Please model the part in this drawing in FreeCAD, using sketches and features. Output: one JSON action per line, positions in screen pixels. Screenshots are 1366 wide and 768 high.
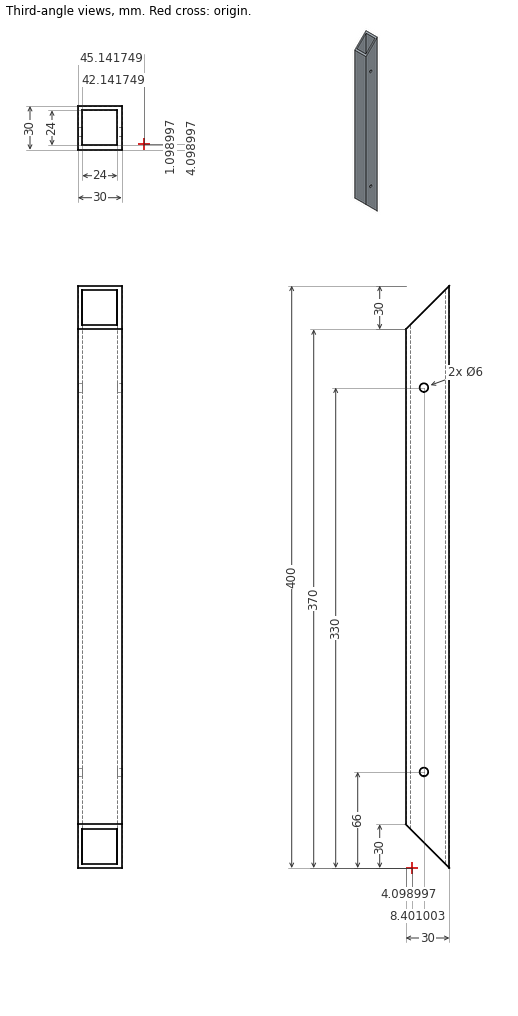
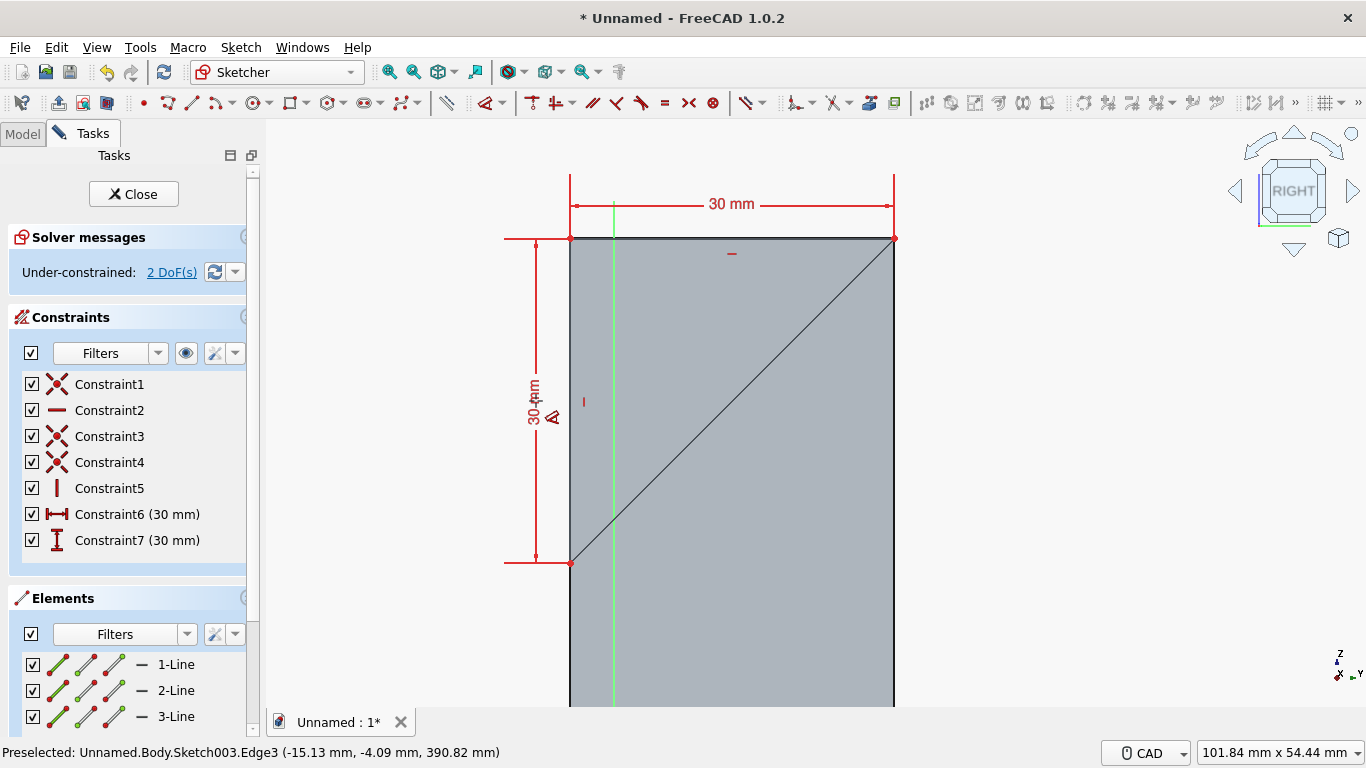
{"action": "left_click", "coordinate": [570, 563]}
{"action": "left_click", "coordinate": [536, 621]}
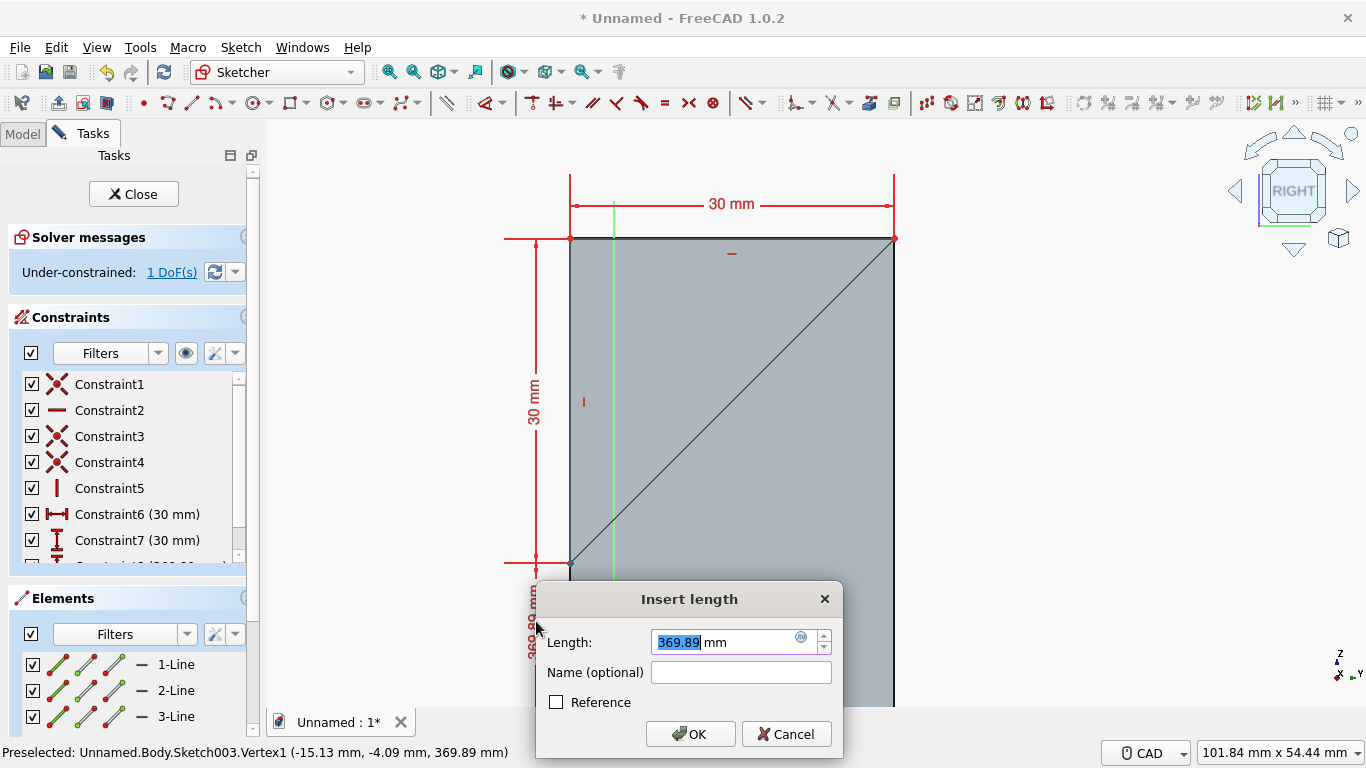
{"action": "type", "text": "370"}
{"action": "key", "text": "Return"}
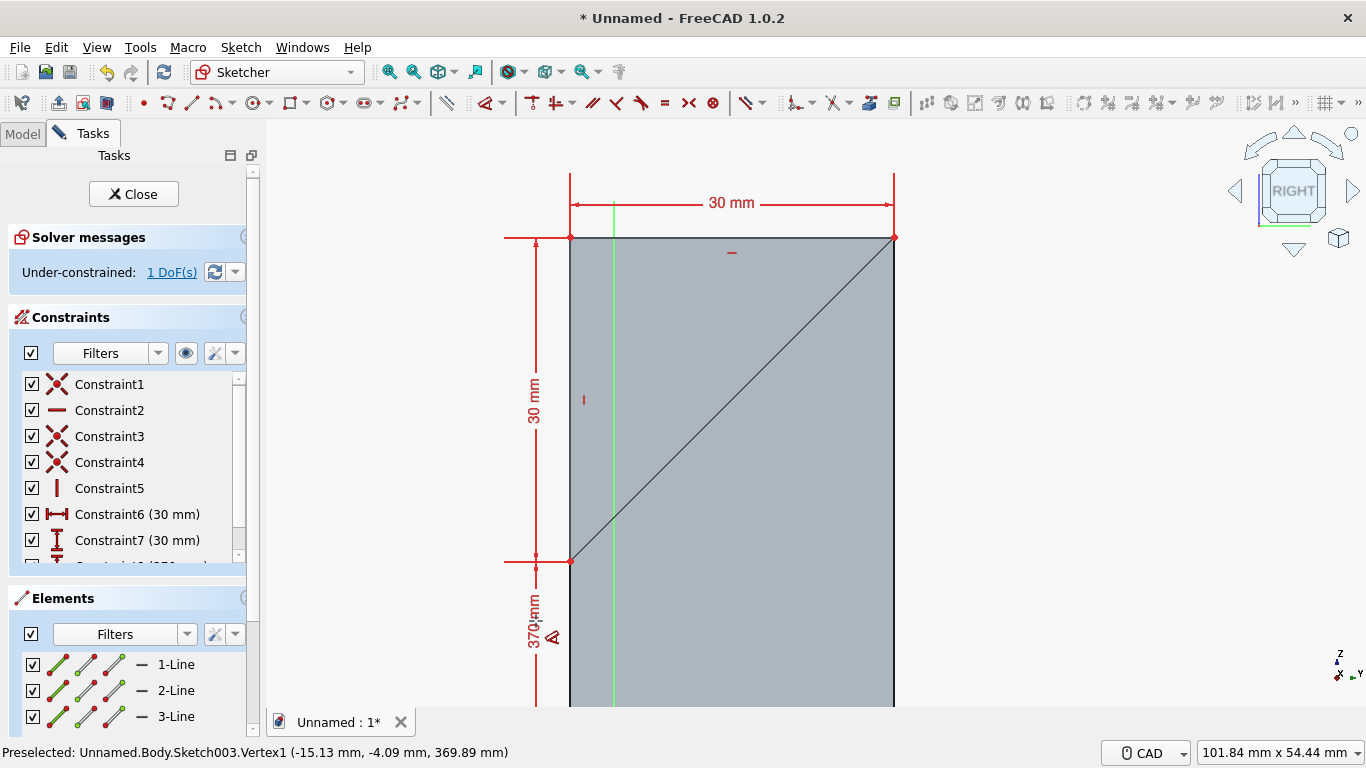
{"action": "left_click", "coordinate": [570, 562]}
{"action": "left_click", "coordinate": [592, 504]}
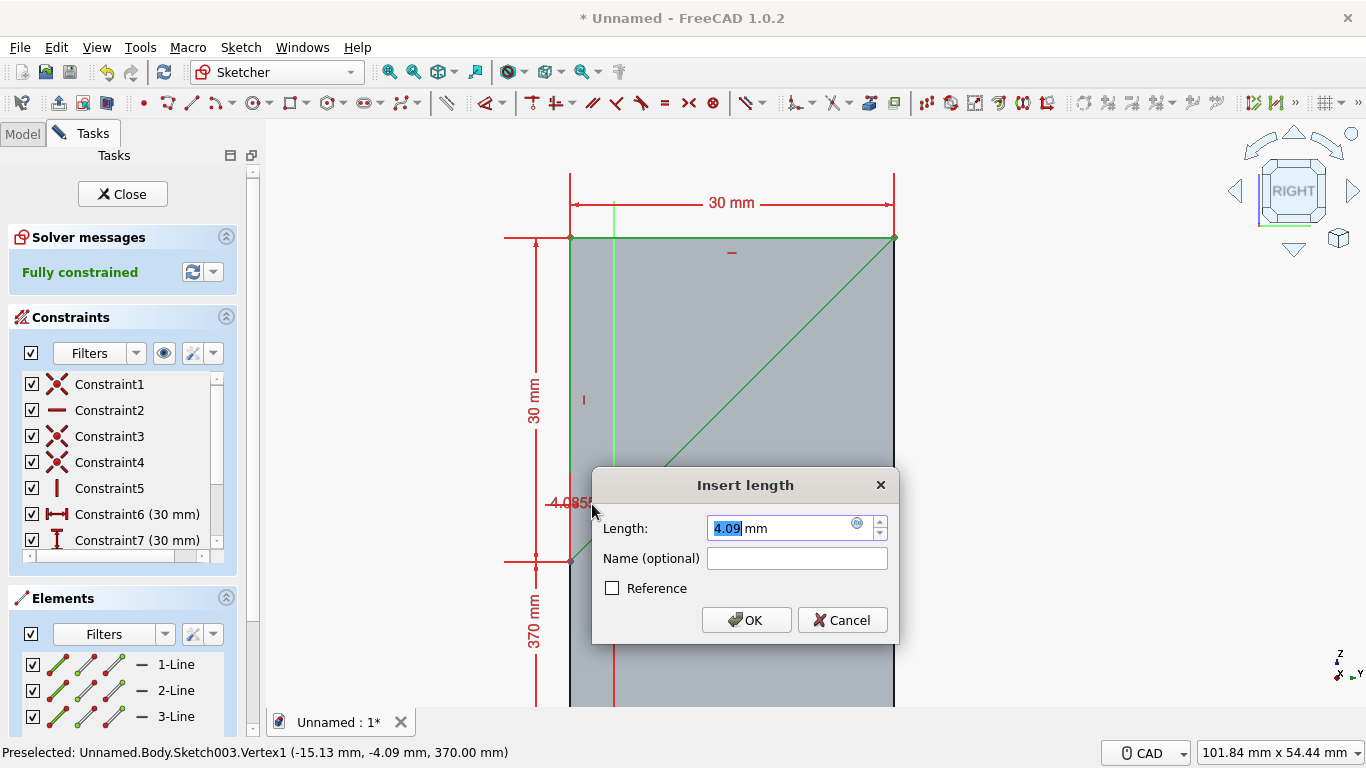
{"action": "type", "text": "4.098997"}
{"action": "key", "text": "Return"}
{"action": "key", "text": "Escape"}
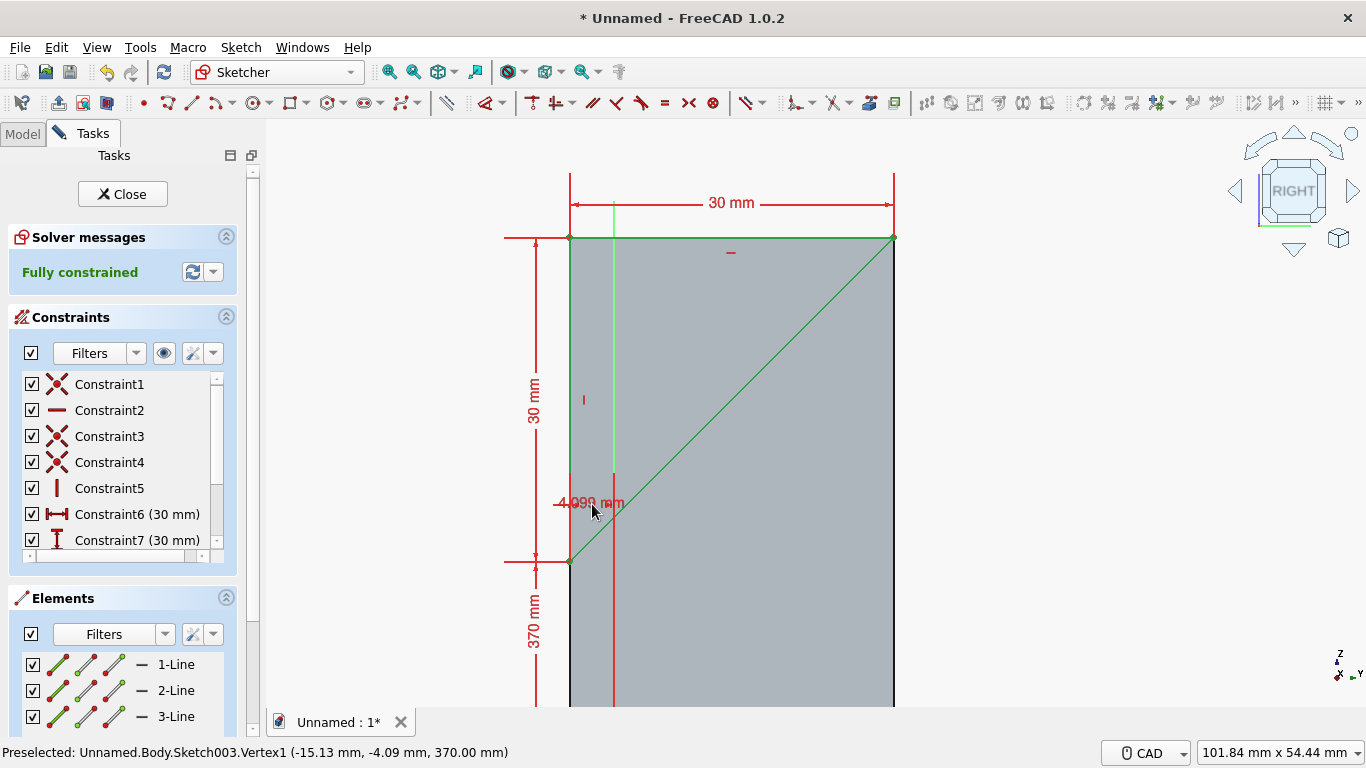
{"action": "left_click", "coordinate": [123, 194]}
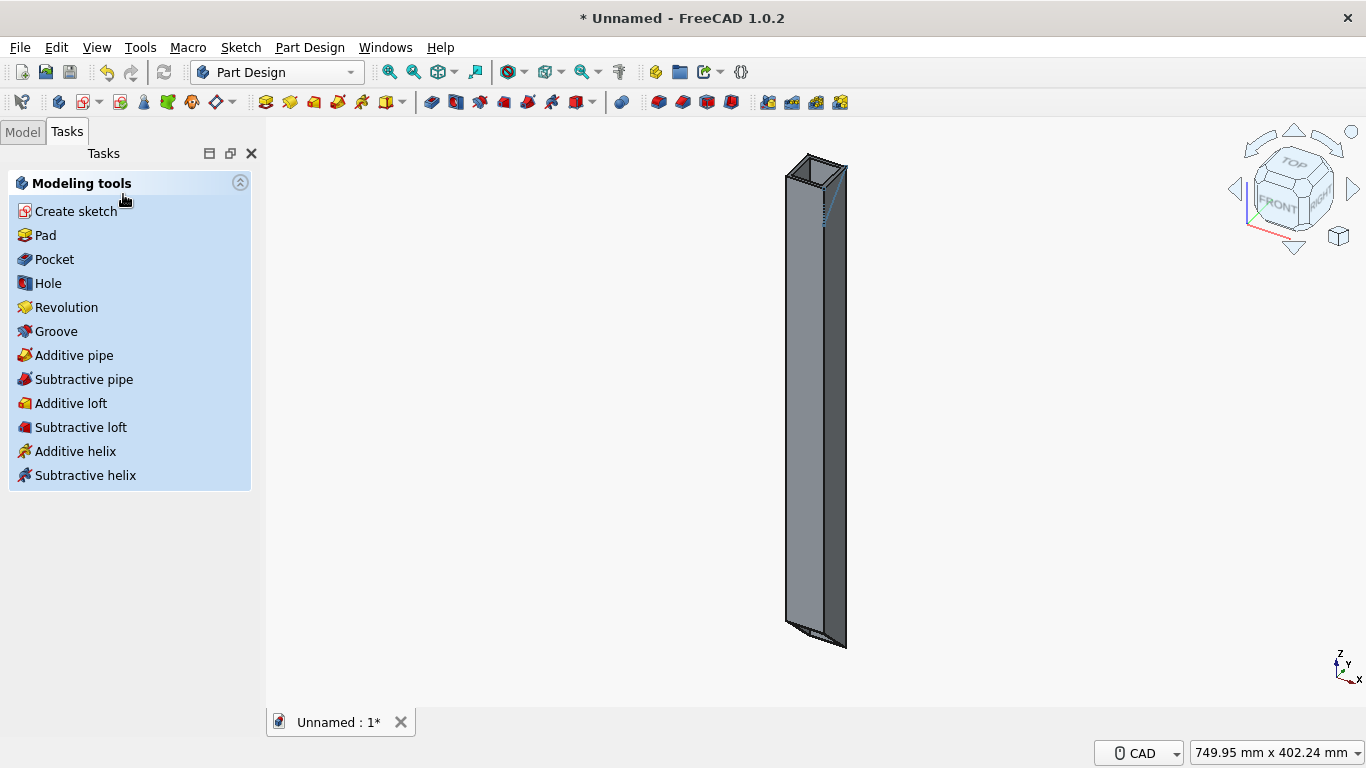
{"action": "left_click", "coordinate": [432, 102]}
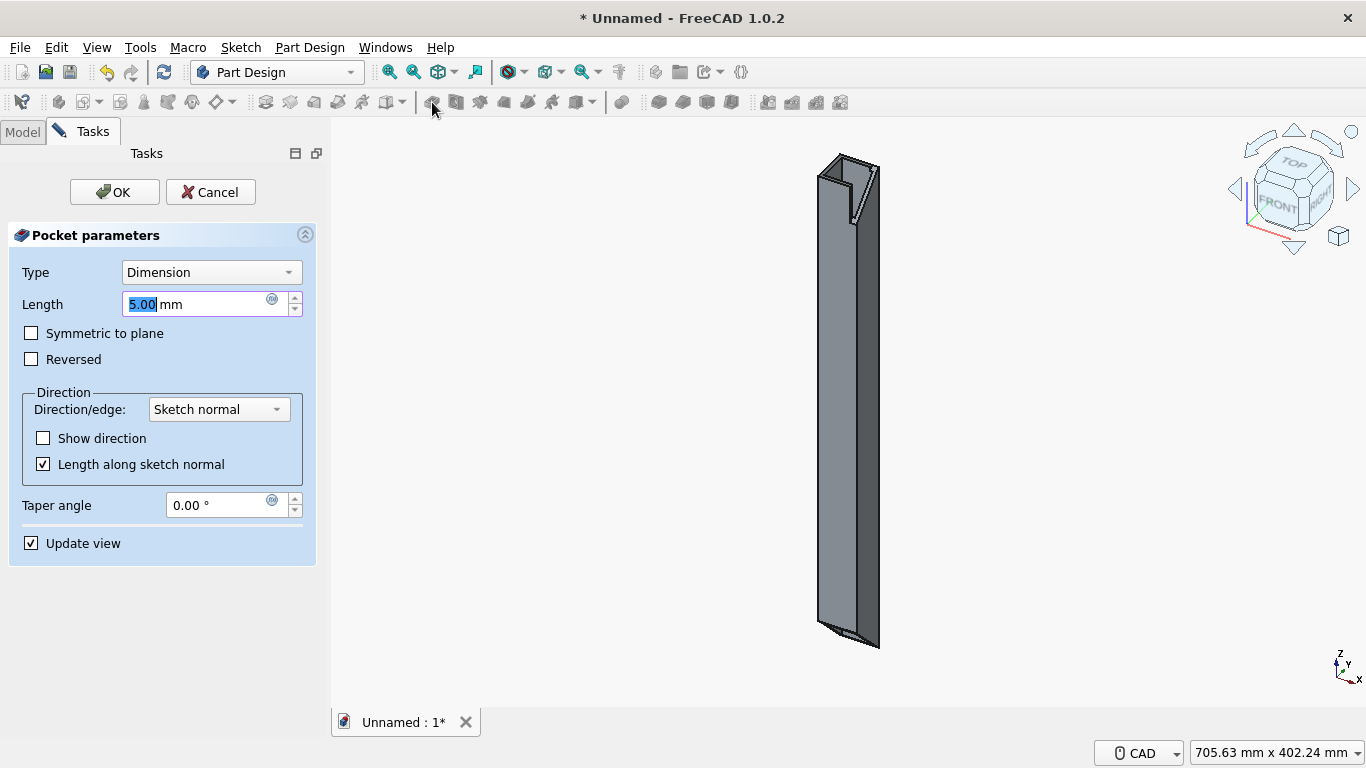
{"action": "left_click", "coordinate": [212, 272]}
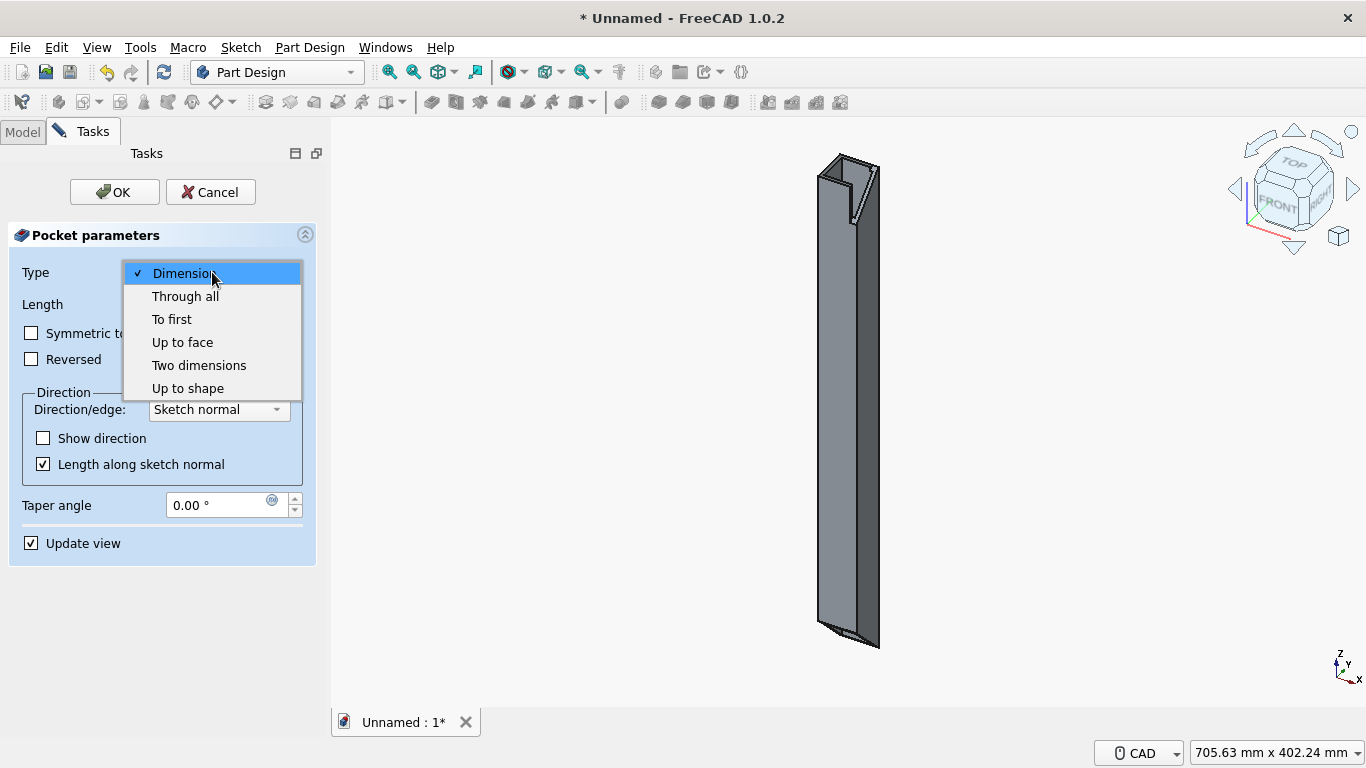
{"action": "left_click", "coordinate": [212, 296]}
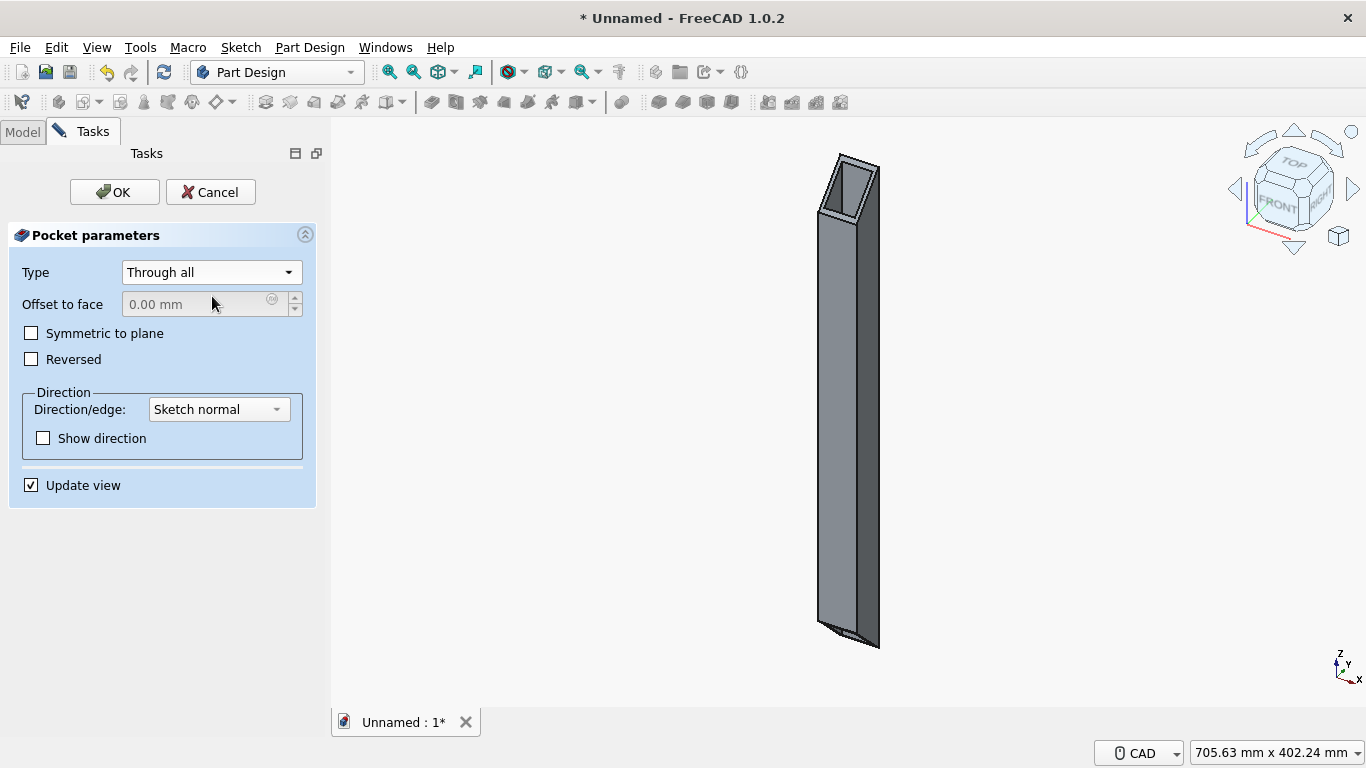
{"action": "left_click", "coordinate": [115, 192]}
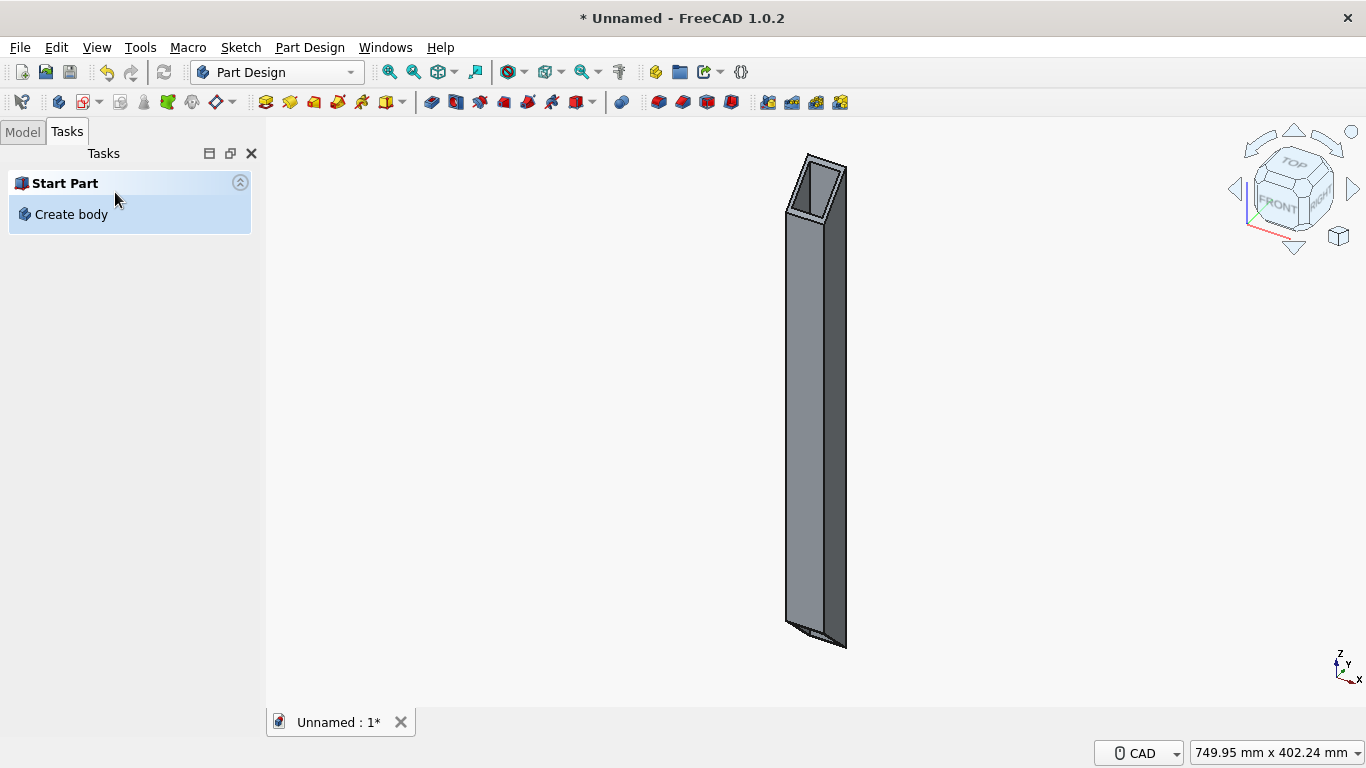
{"action": "left_click", "coordinate": [835, 280]}